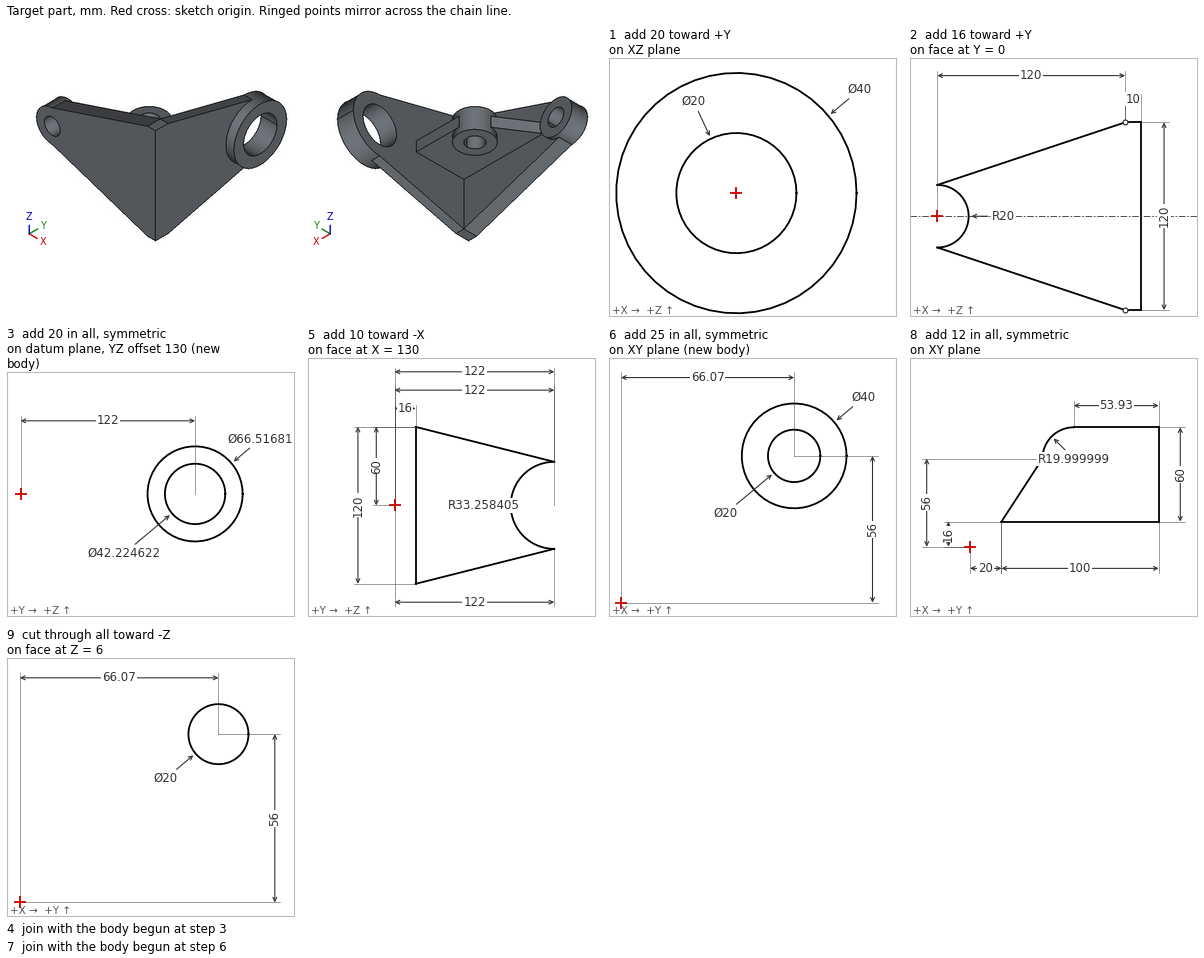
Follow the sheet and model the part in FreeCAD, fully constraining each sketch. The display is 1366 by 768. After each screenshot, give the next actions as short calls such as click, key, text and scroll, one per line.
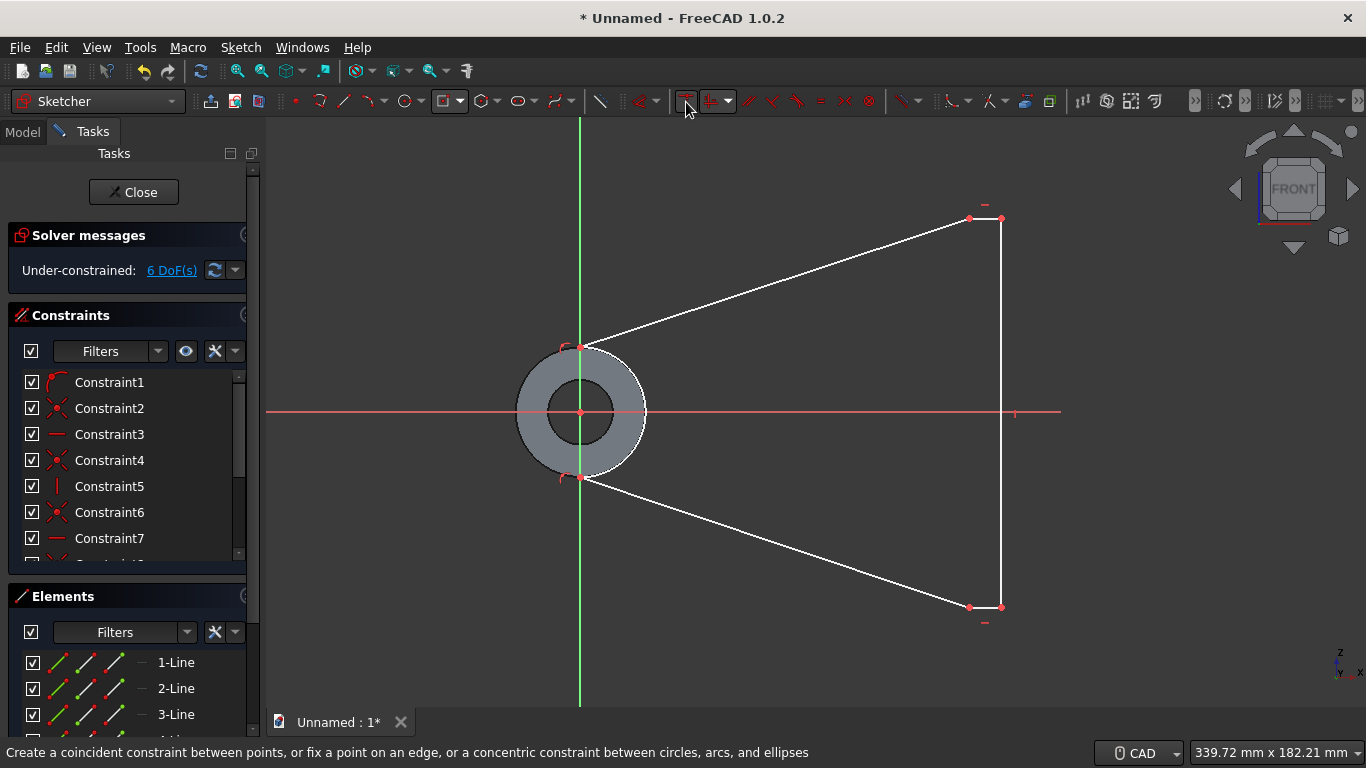
click(969, 219)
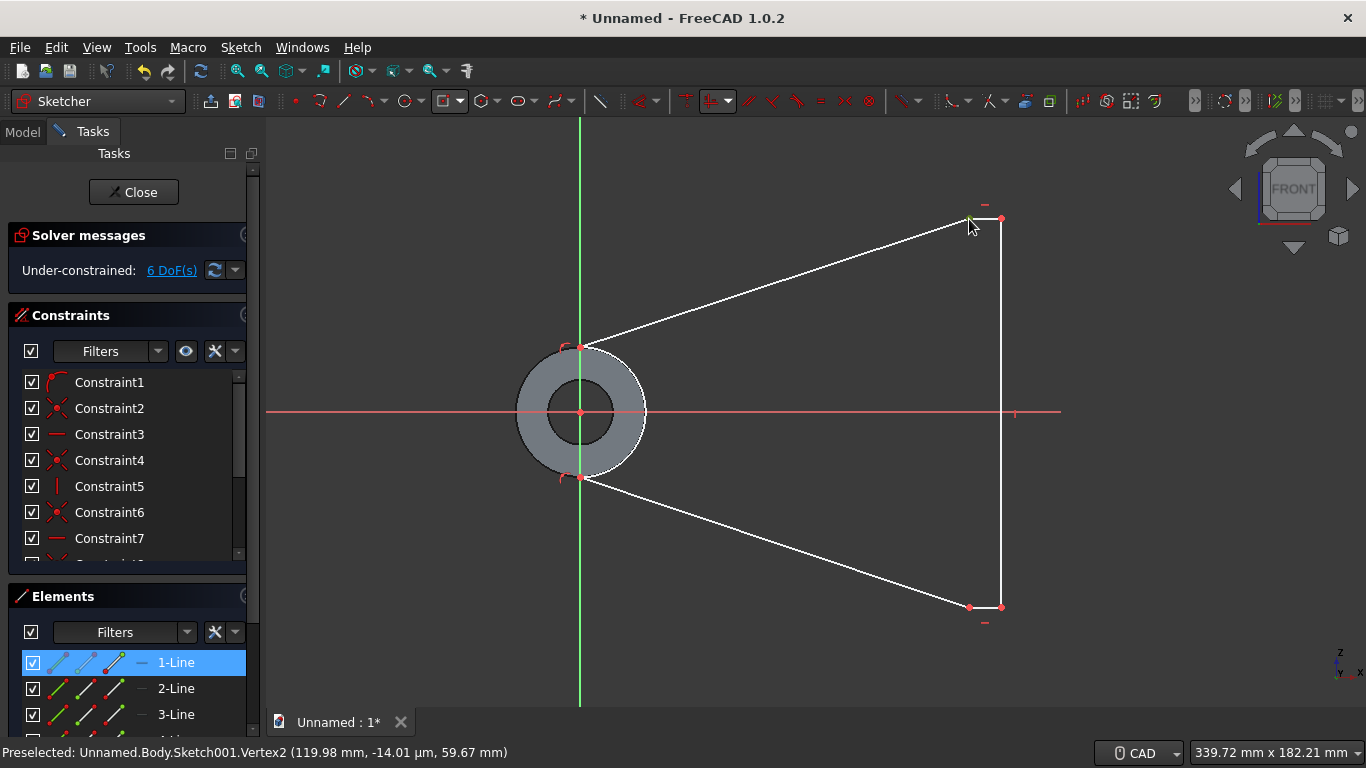
click(969, 608)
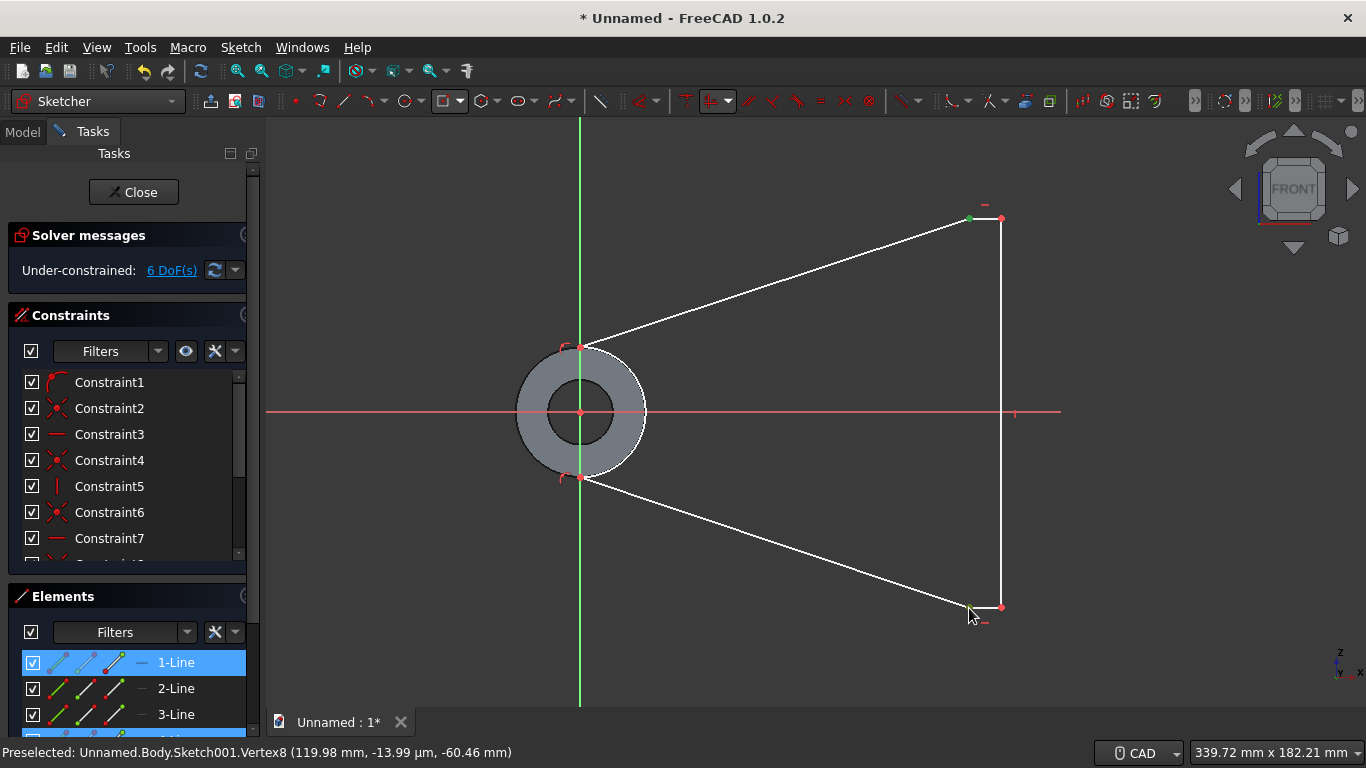
click(359, 412)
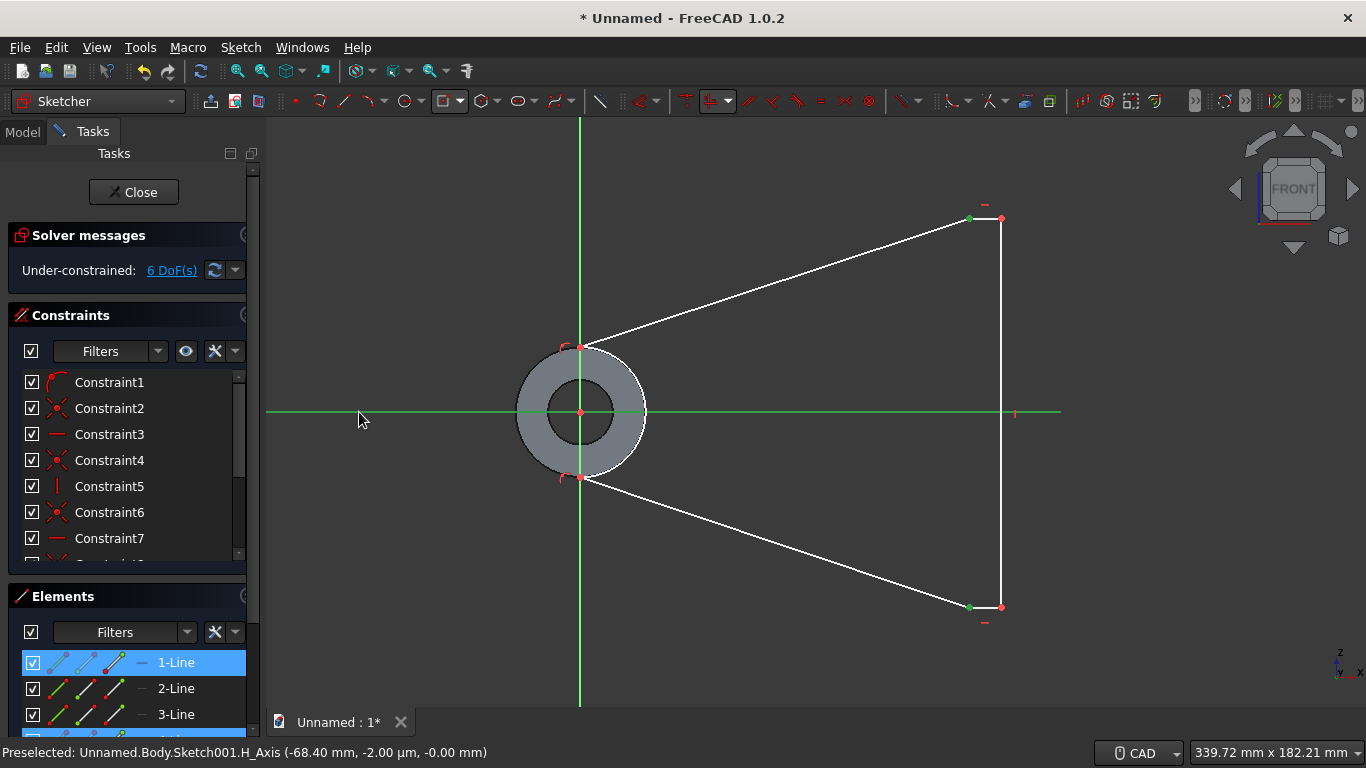
click(846, 102)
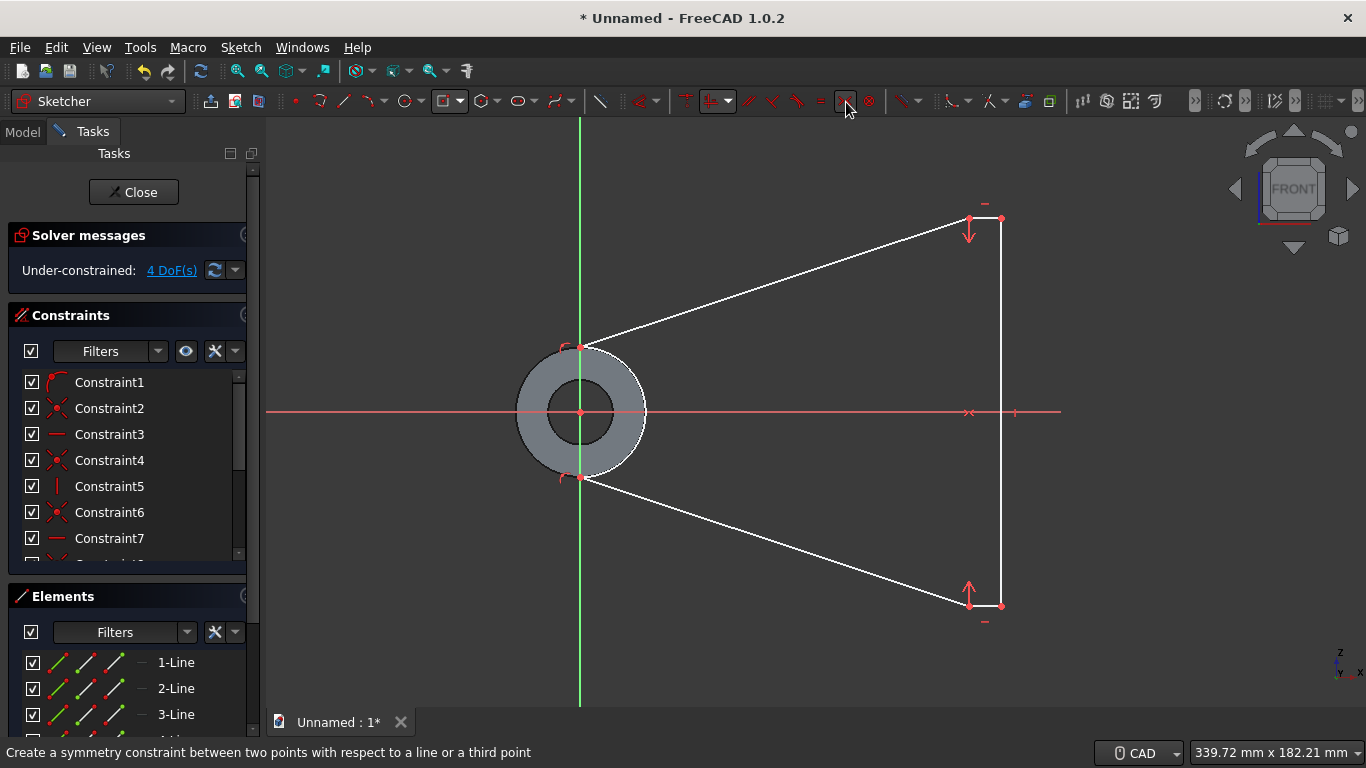
click(640, 102)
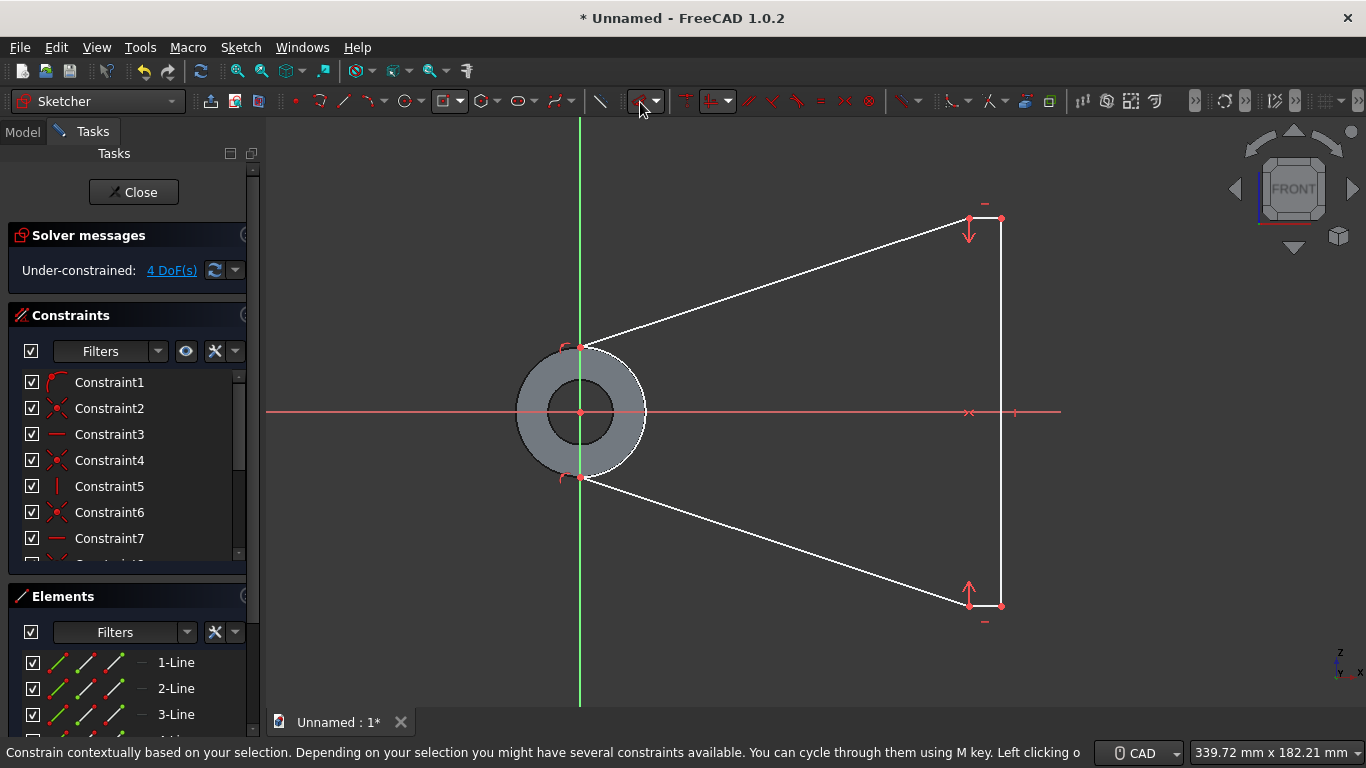
click(633, 451)
click(659, 470)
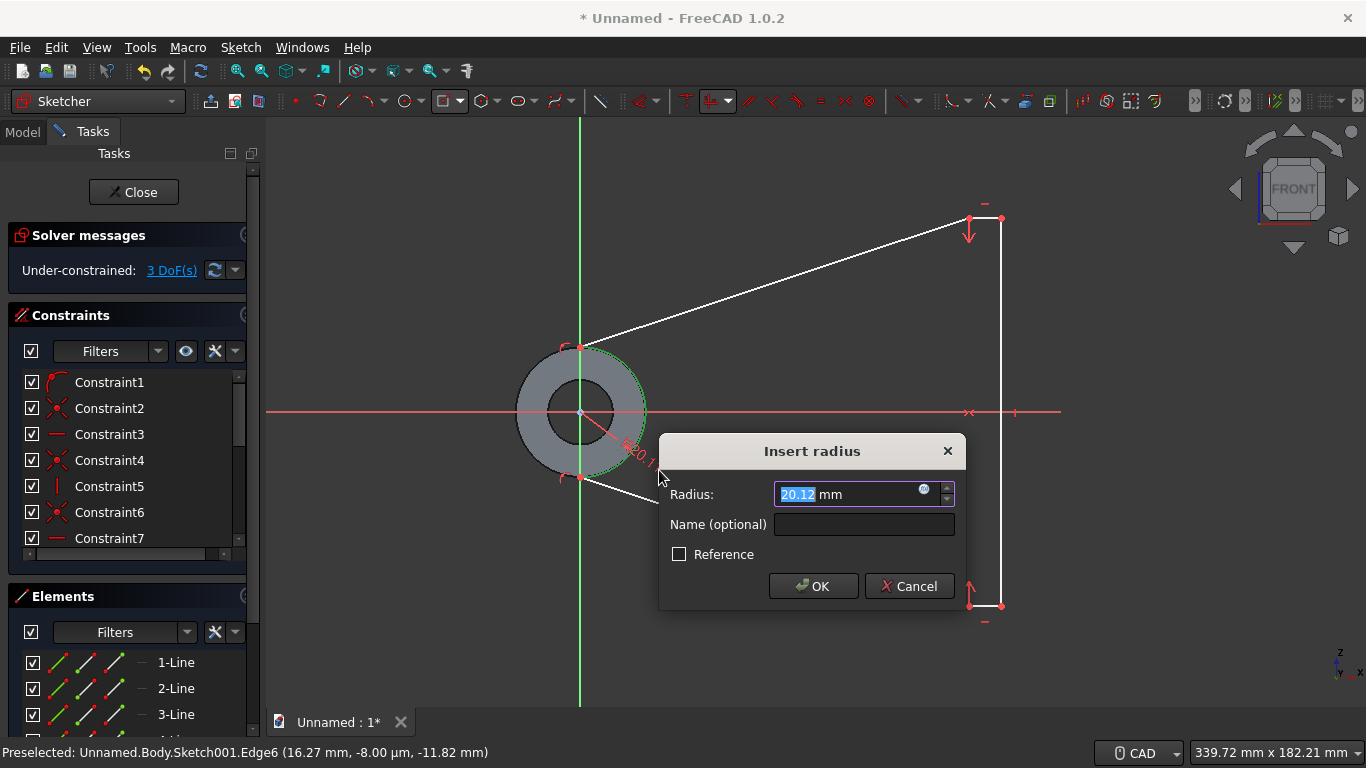
text(20)
key(Return)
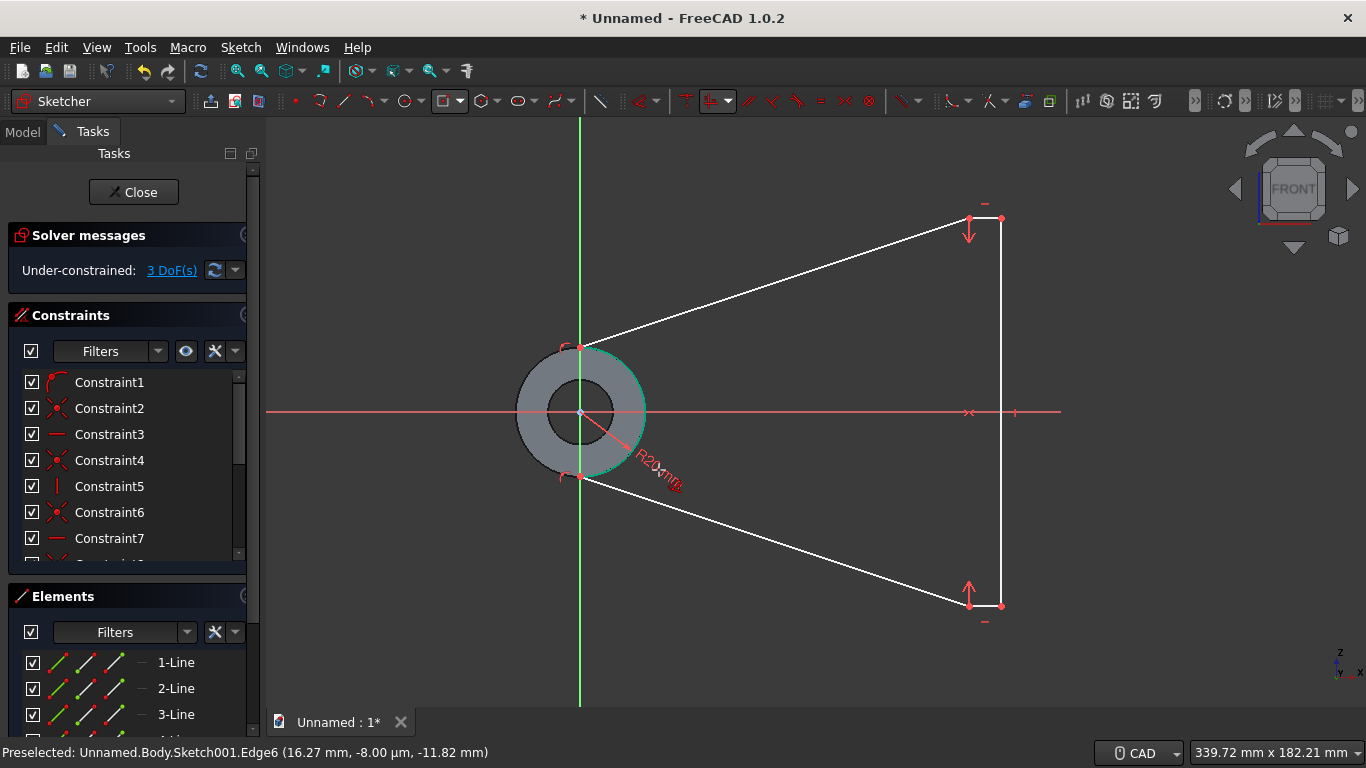
scroll(979, 218, up, 2)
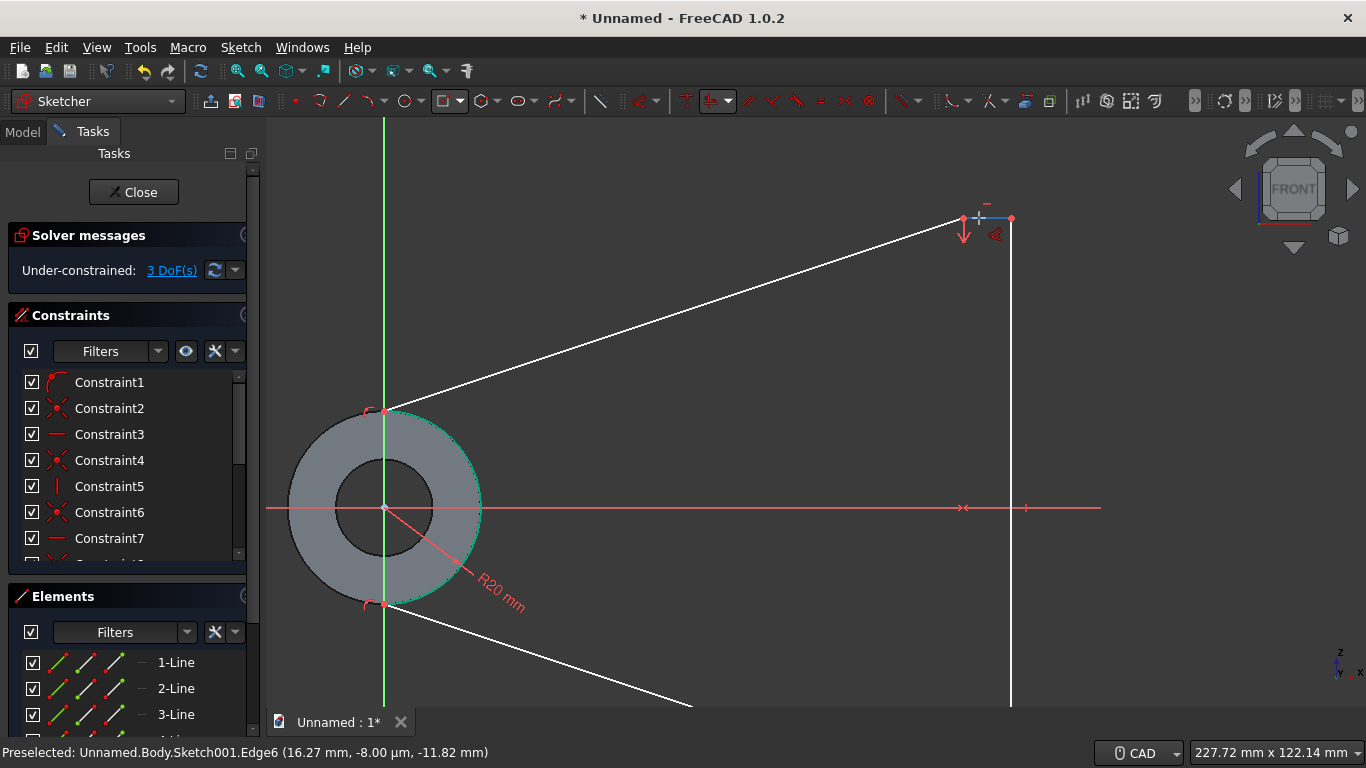
click(978, 218)
click(988, 184)